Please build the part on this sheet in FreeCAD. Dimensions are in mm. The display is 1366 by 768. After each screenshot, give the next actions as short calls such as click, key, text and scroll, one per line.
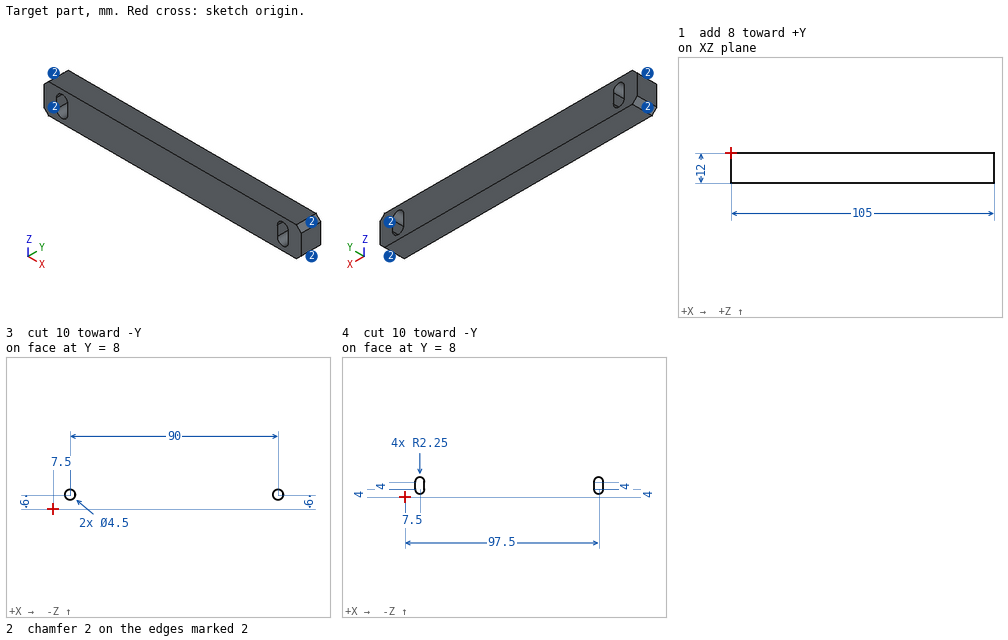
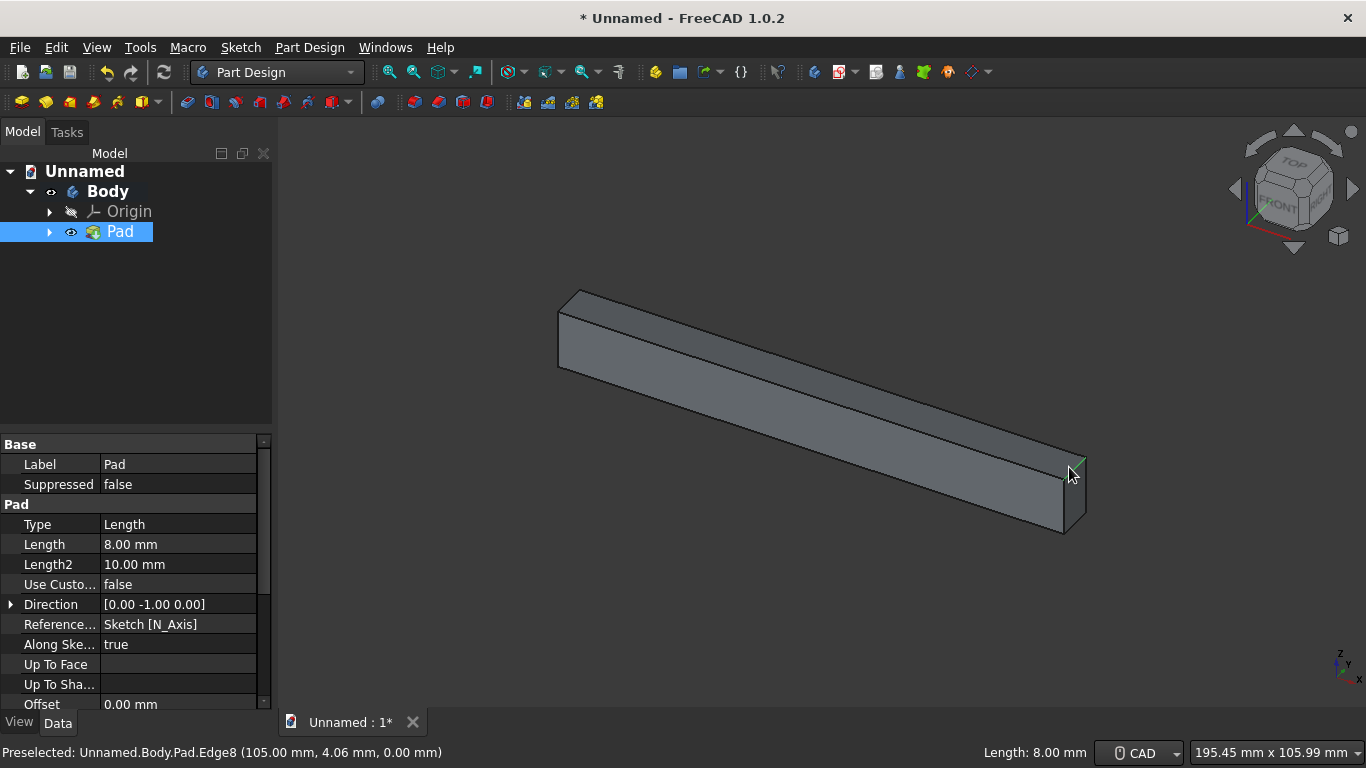
key(0)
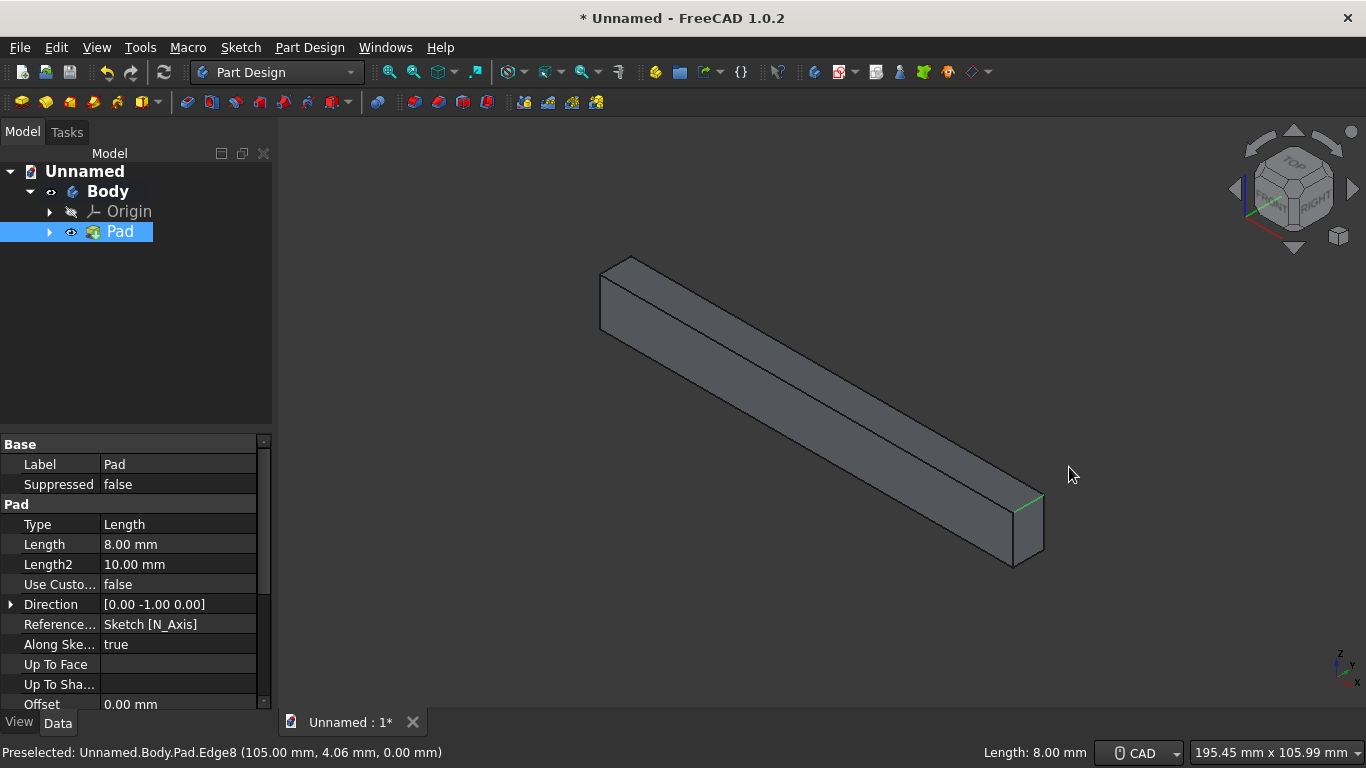
key(2)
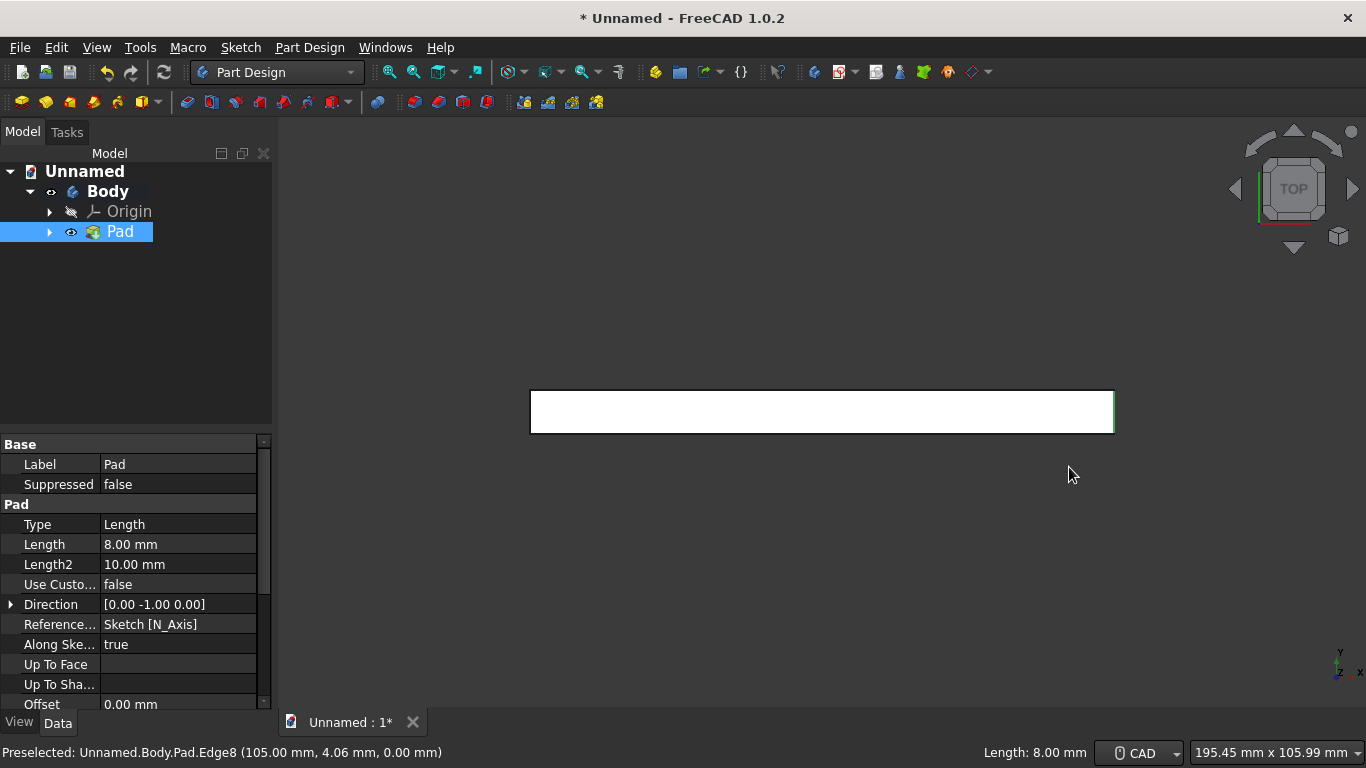
key(1)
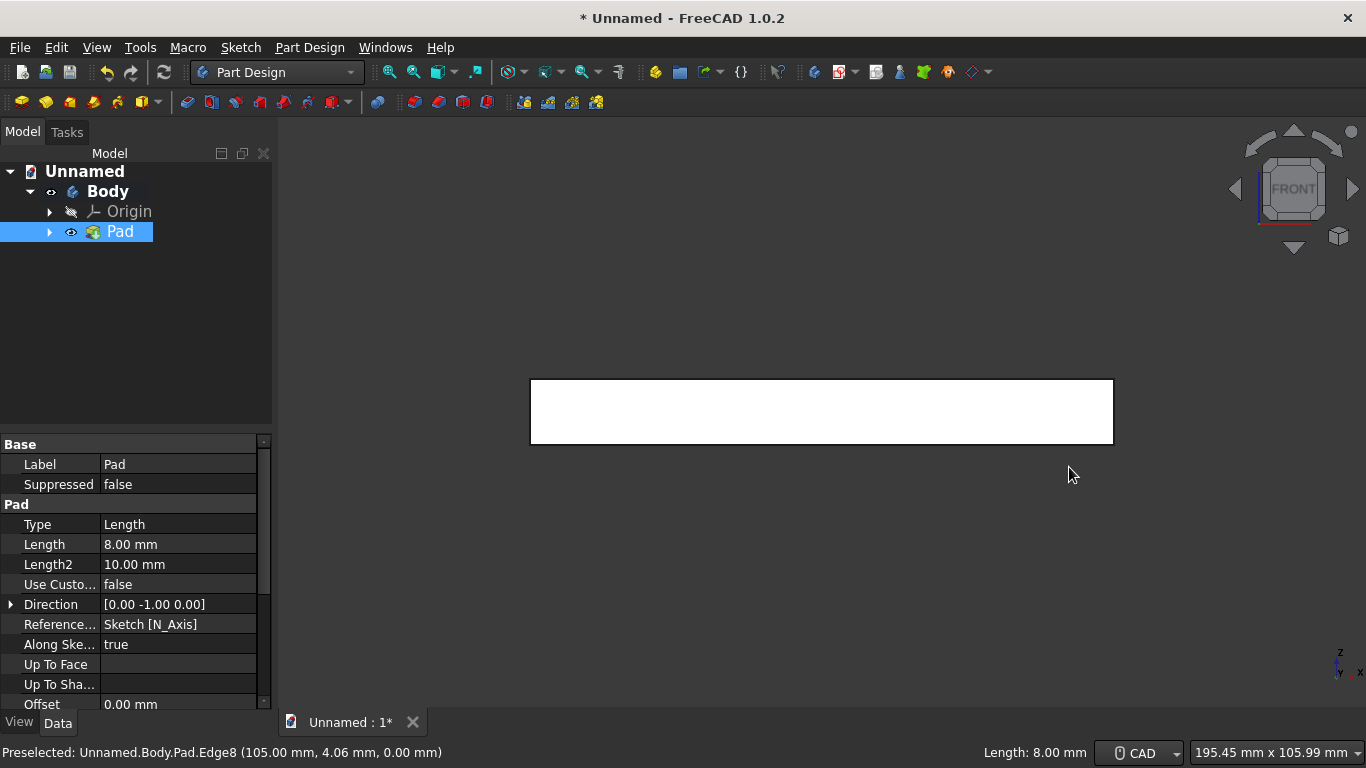
key(3)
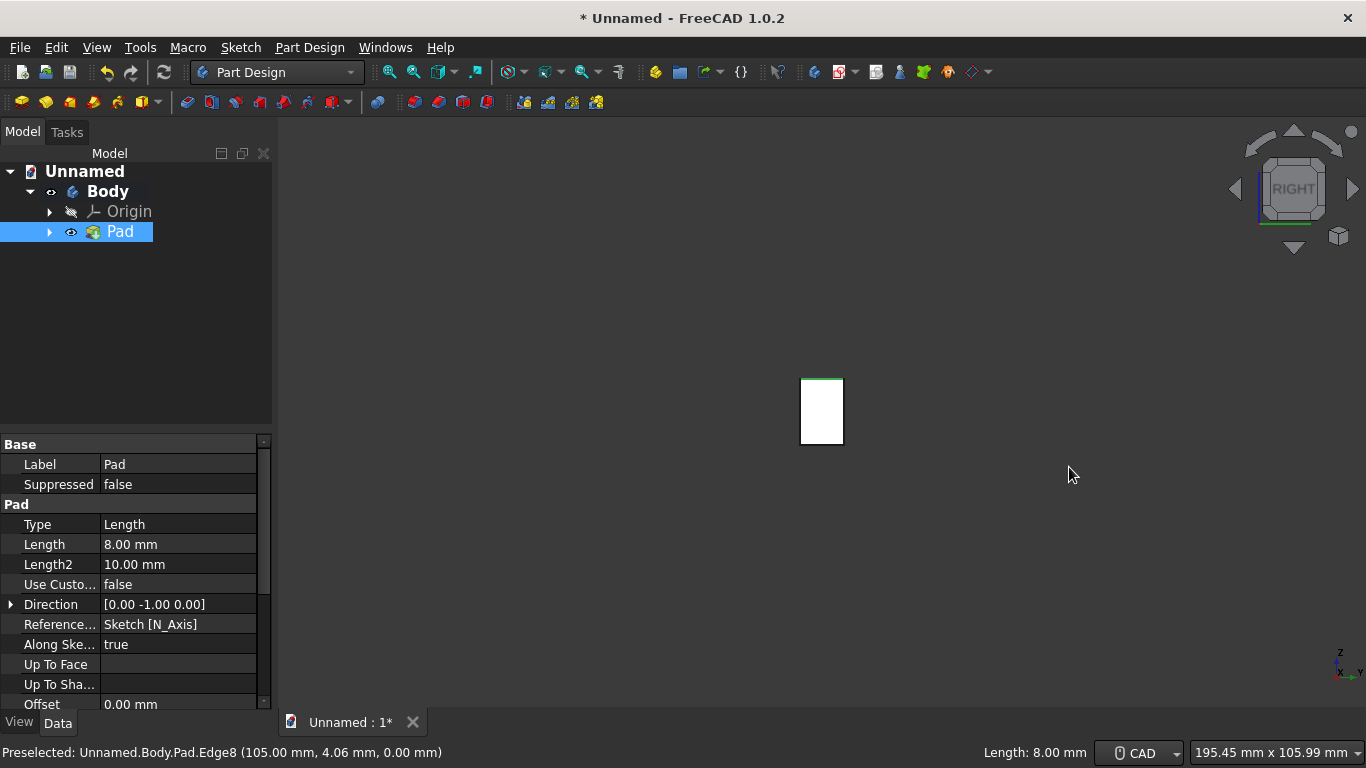
click(390, 72)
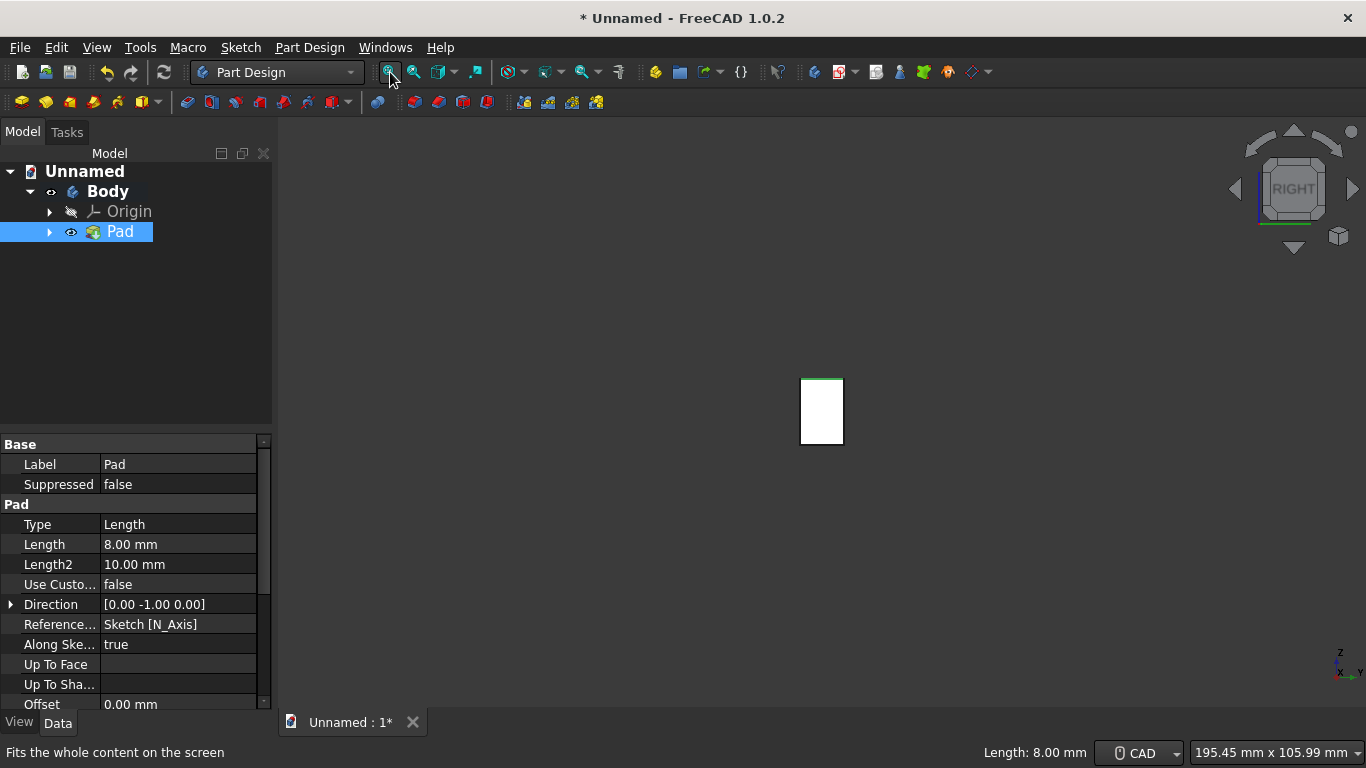
click(822, 444, ctrl)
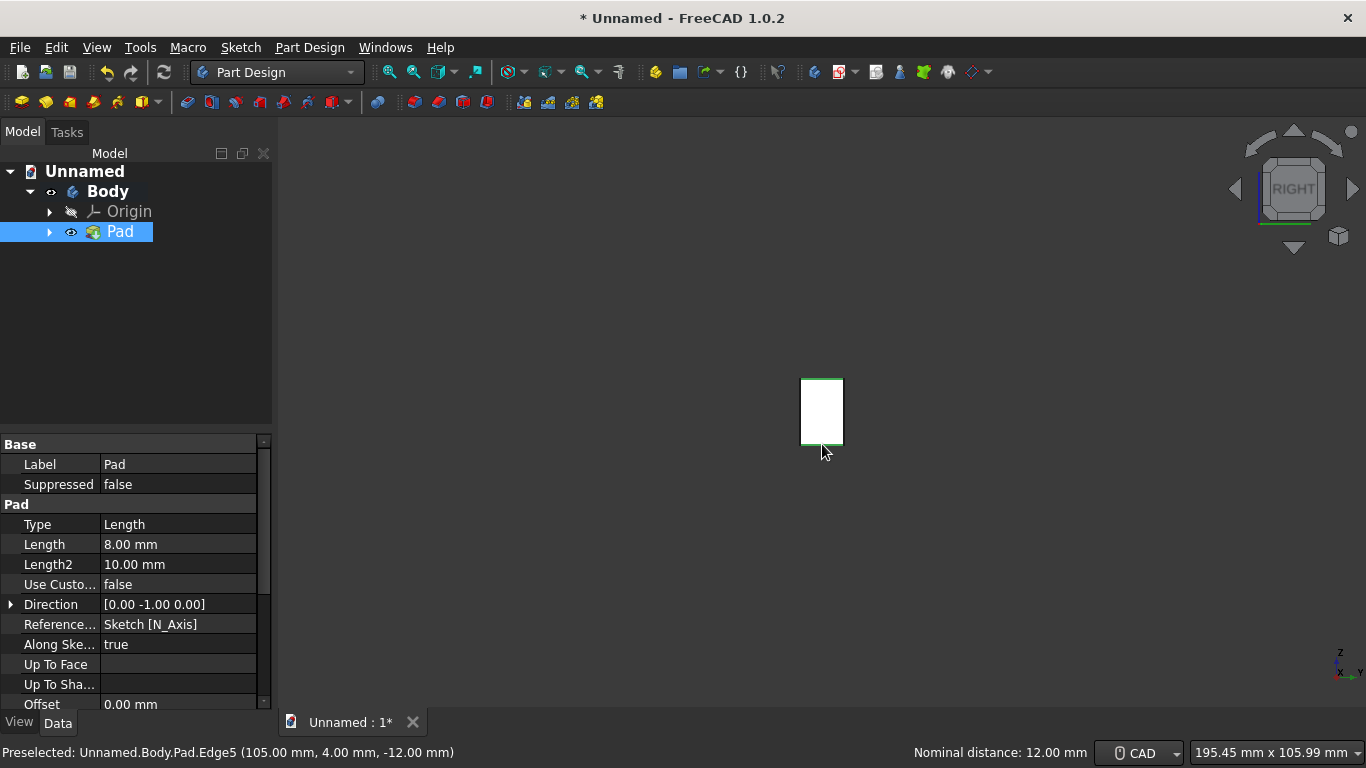
key(5)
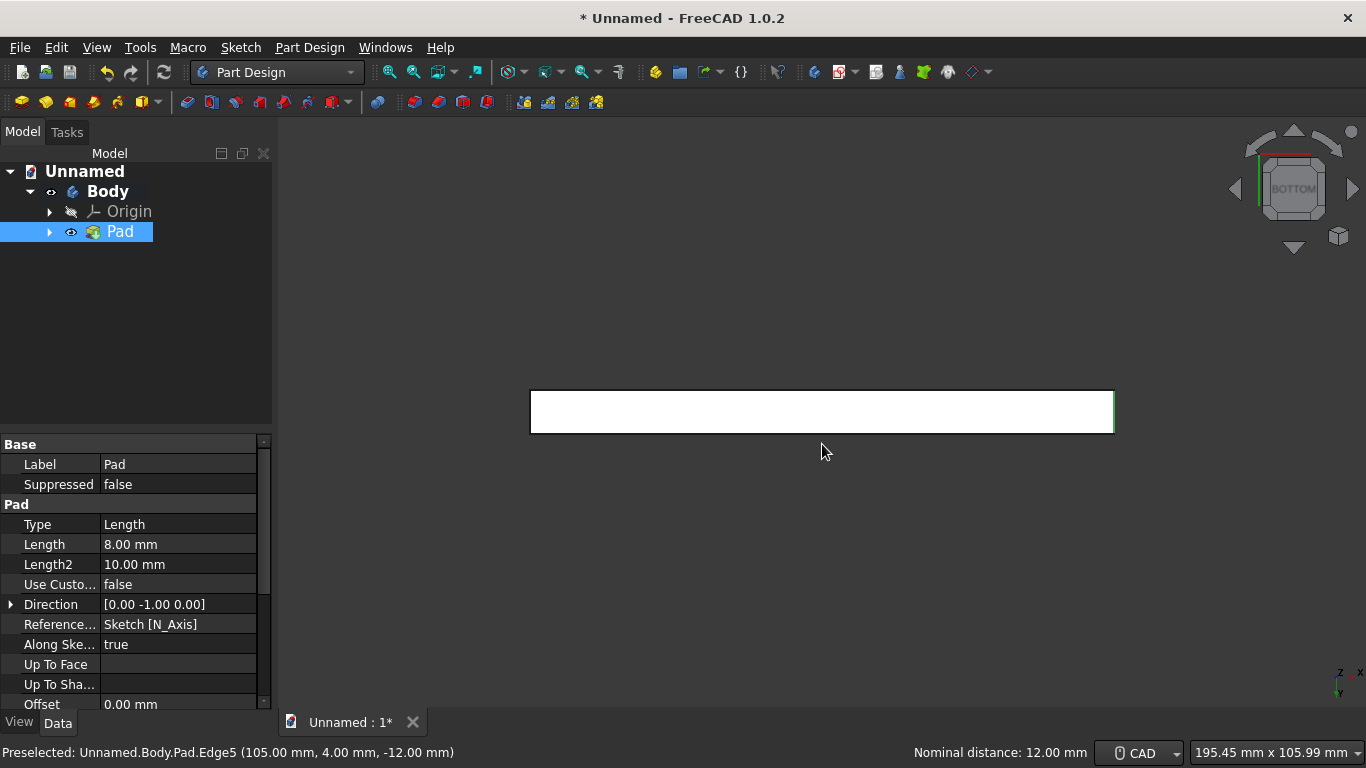
click(530, 411, ctrl)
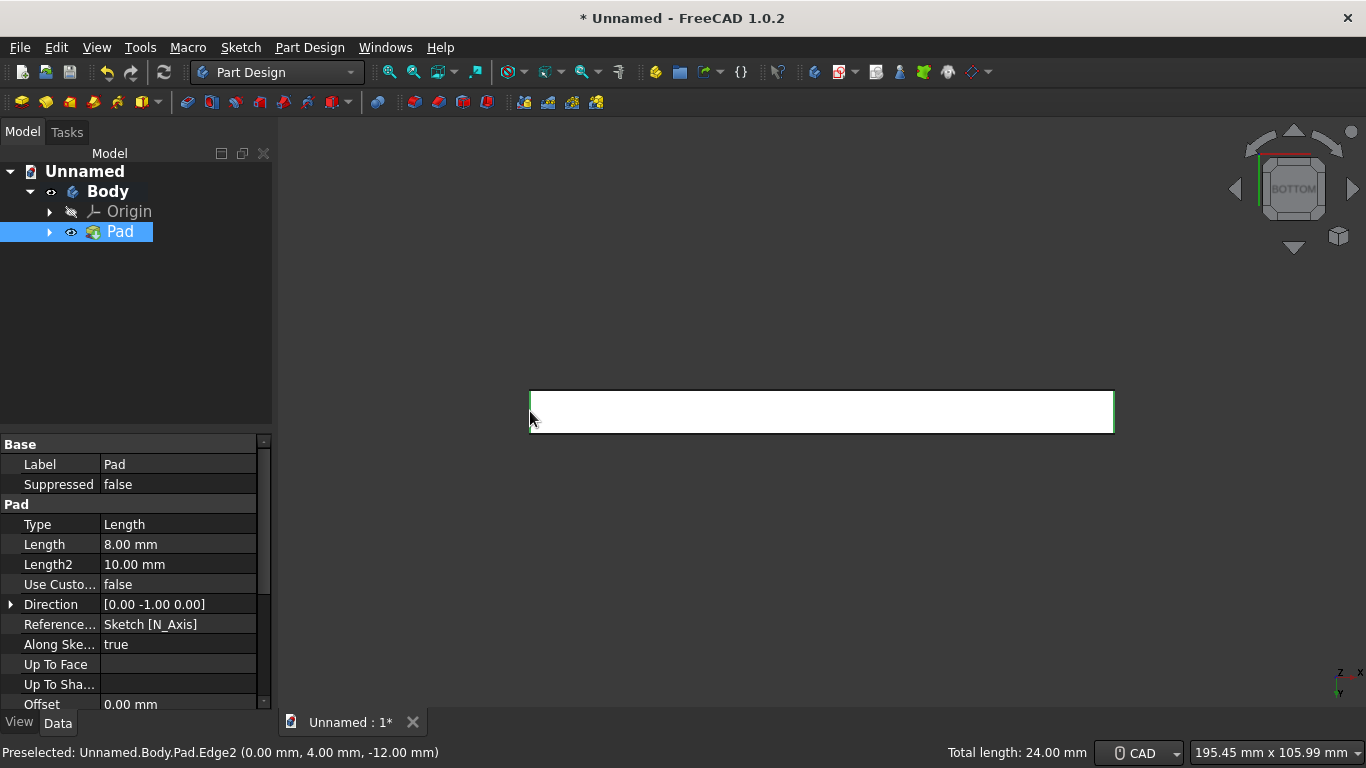
key(4)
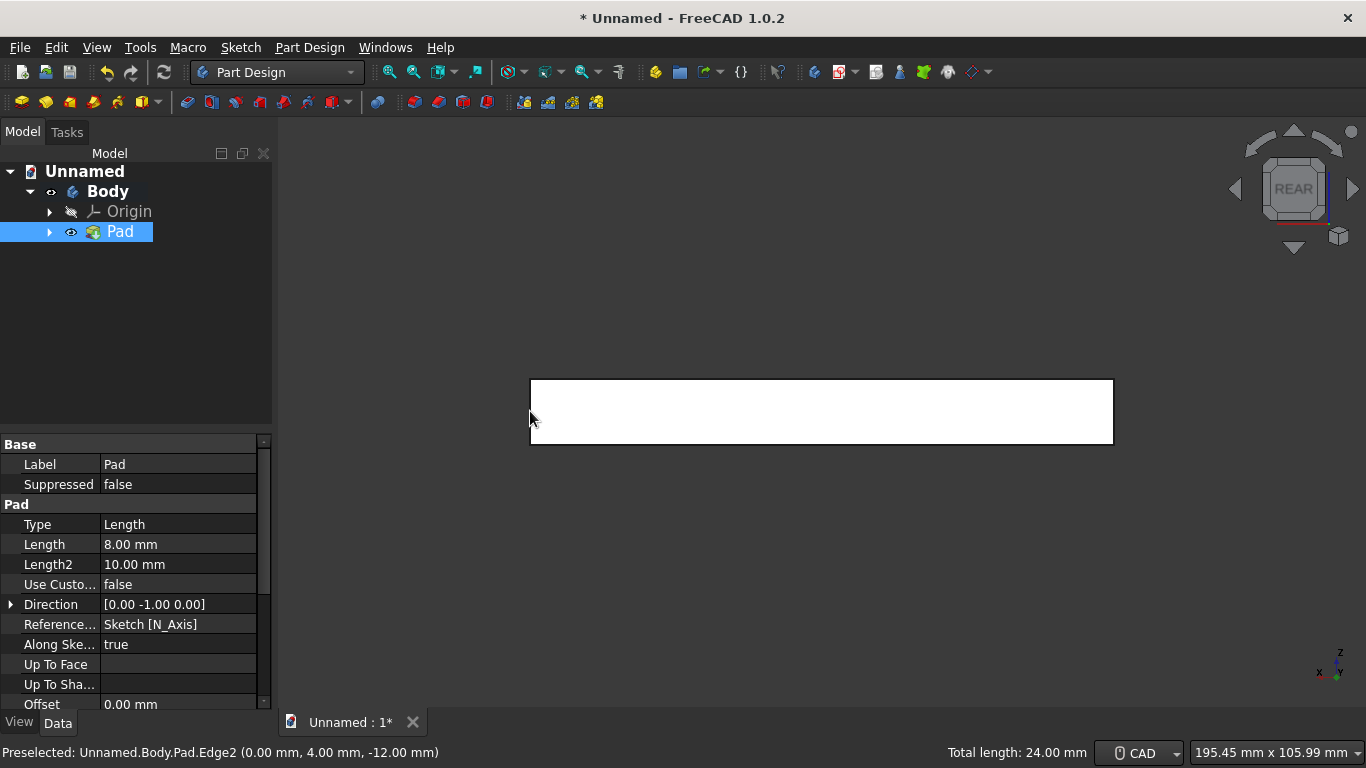
key(6)